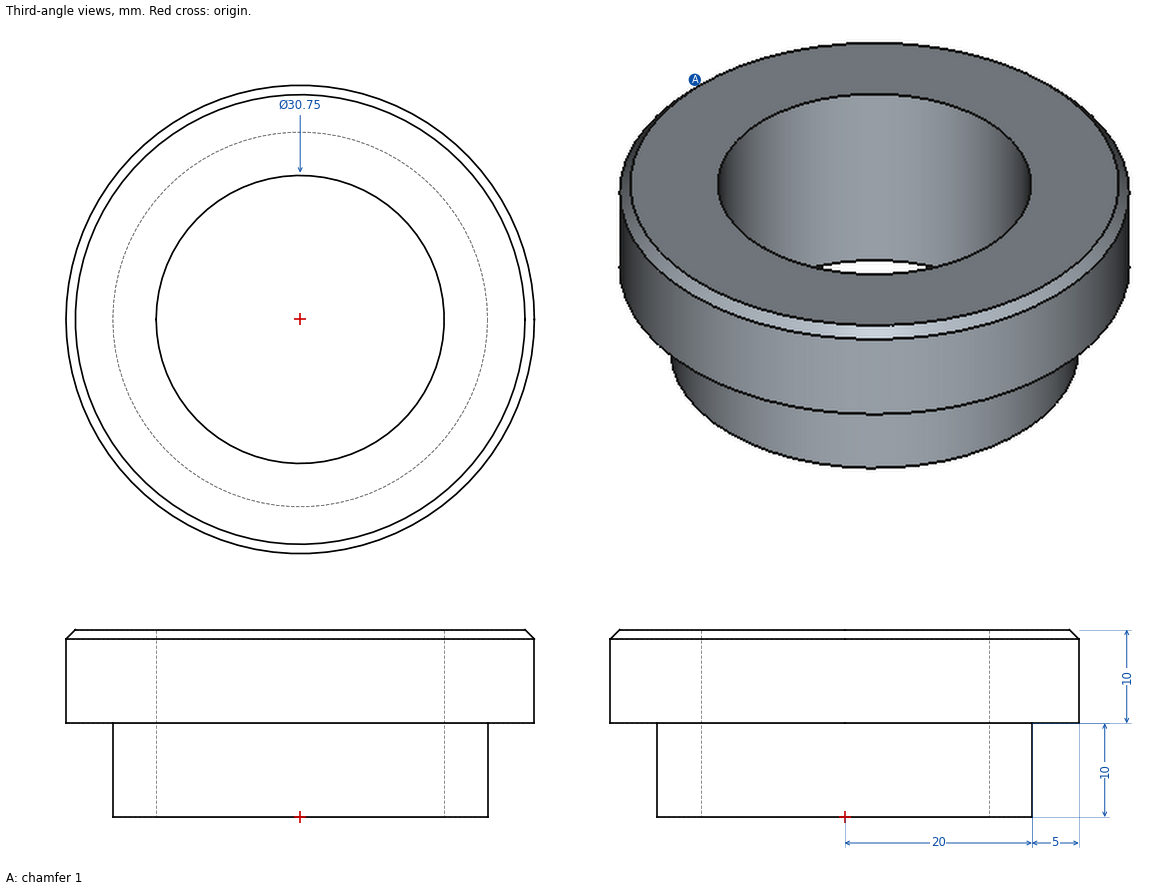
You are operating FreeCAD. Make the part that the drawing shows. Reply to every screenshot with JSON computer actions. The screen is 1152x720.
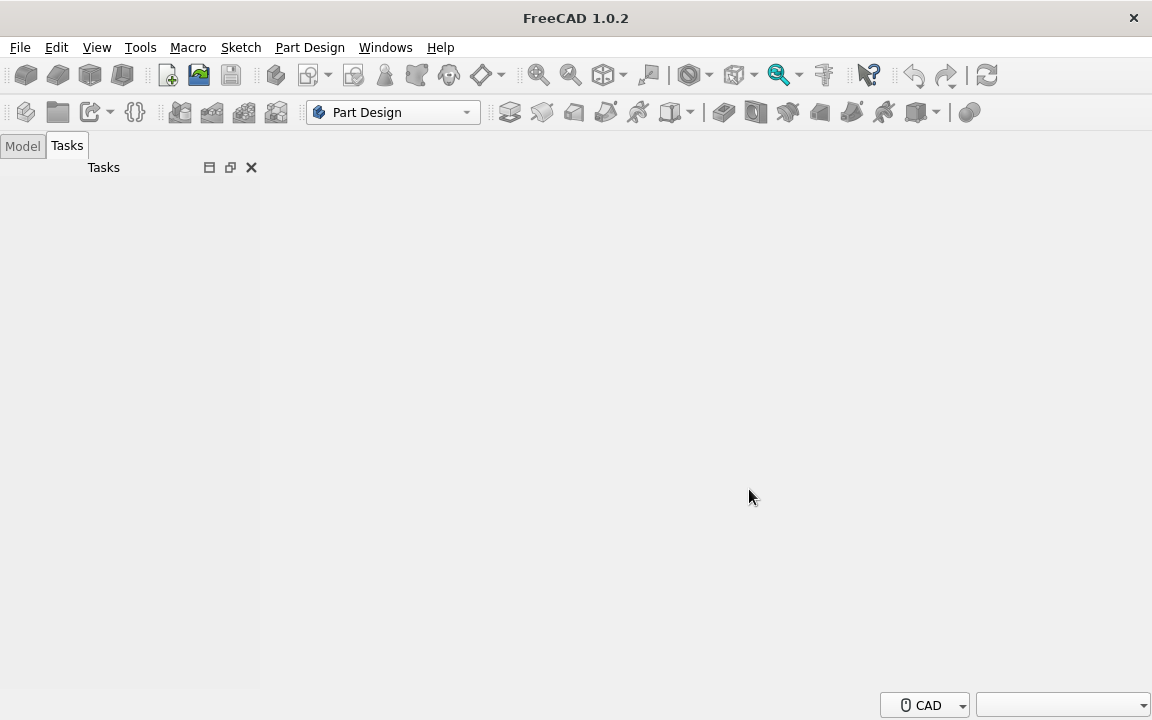
{"action": "key", "text": "ctrl+n"}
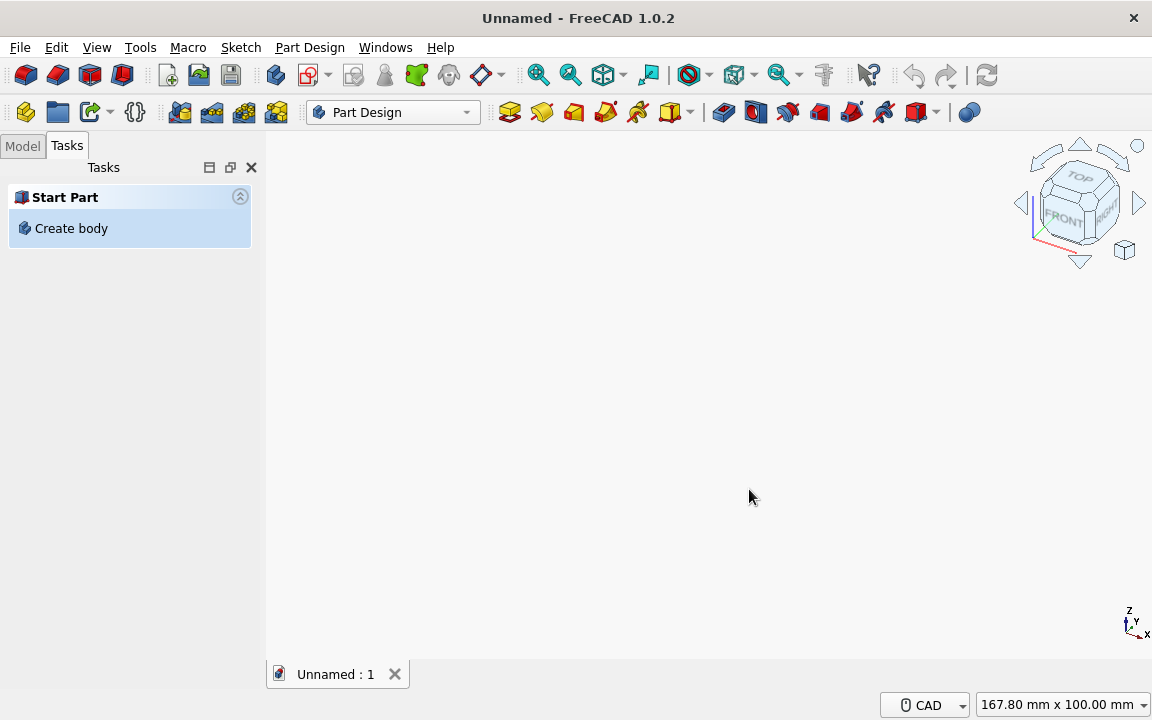
{"action": "left_click", "coordinate": [308, 76]}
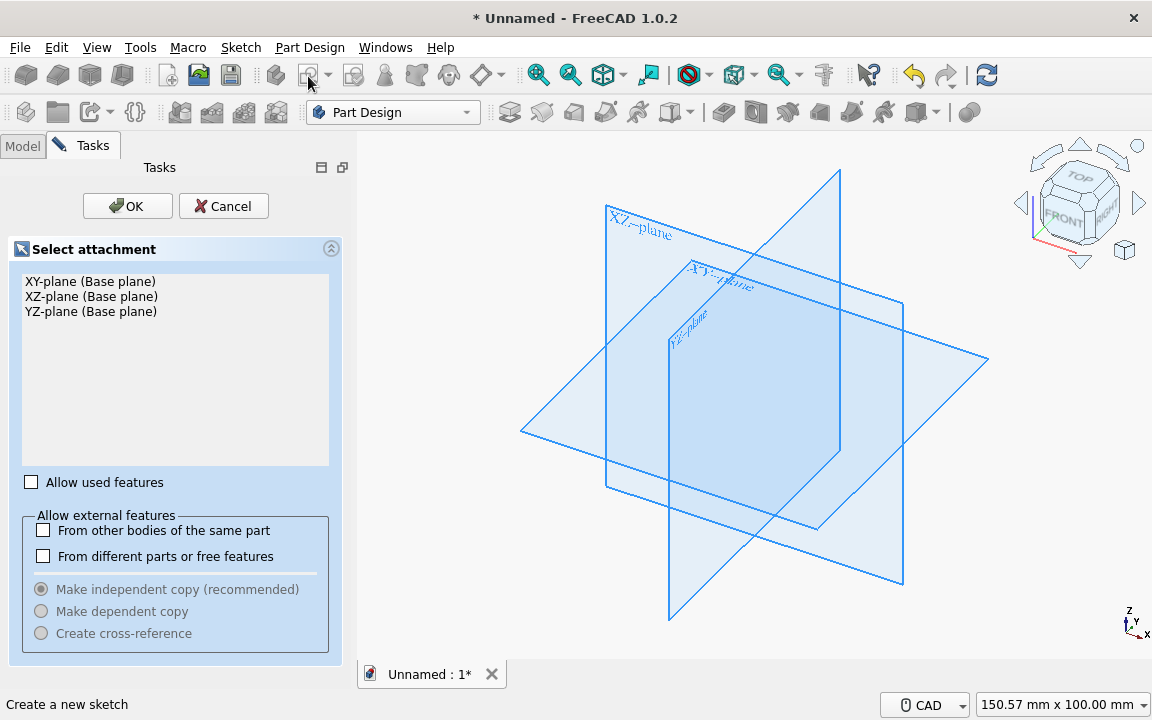
{"action": "left_click", "coordinate": [82, 312]}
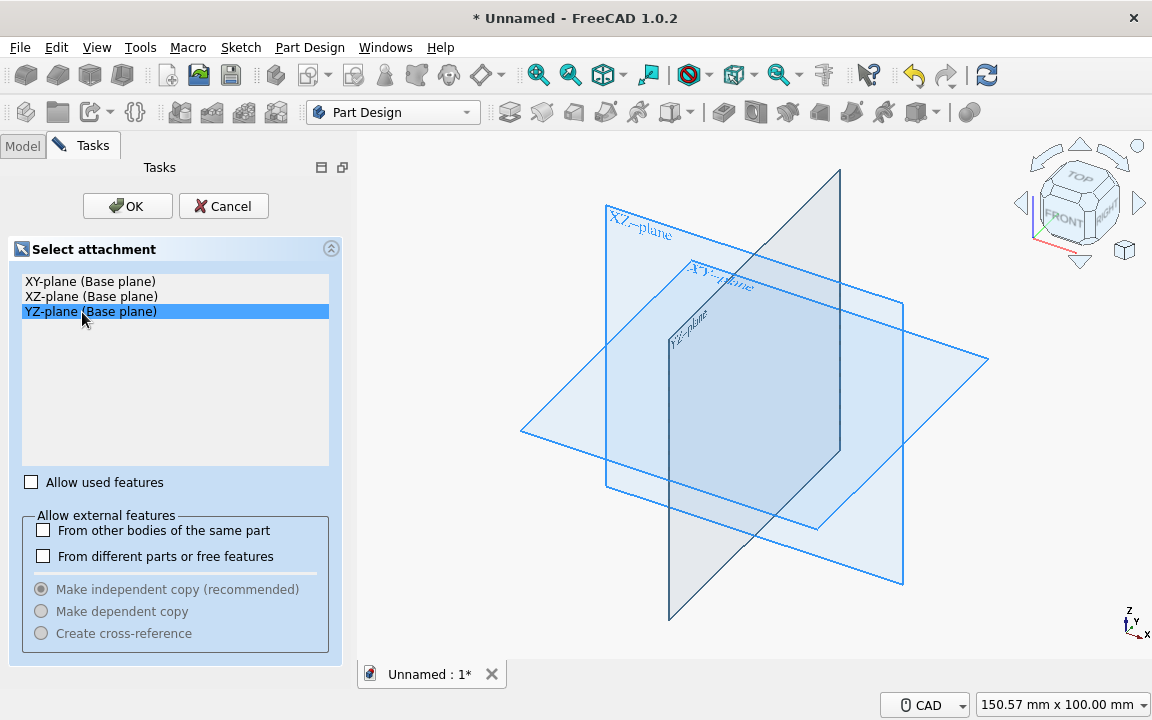
{"action": "left_click", "coordinate": [128, 206]}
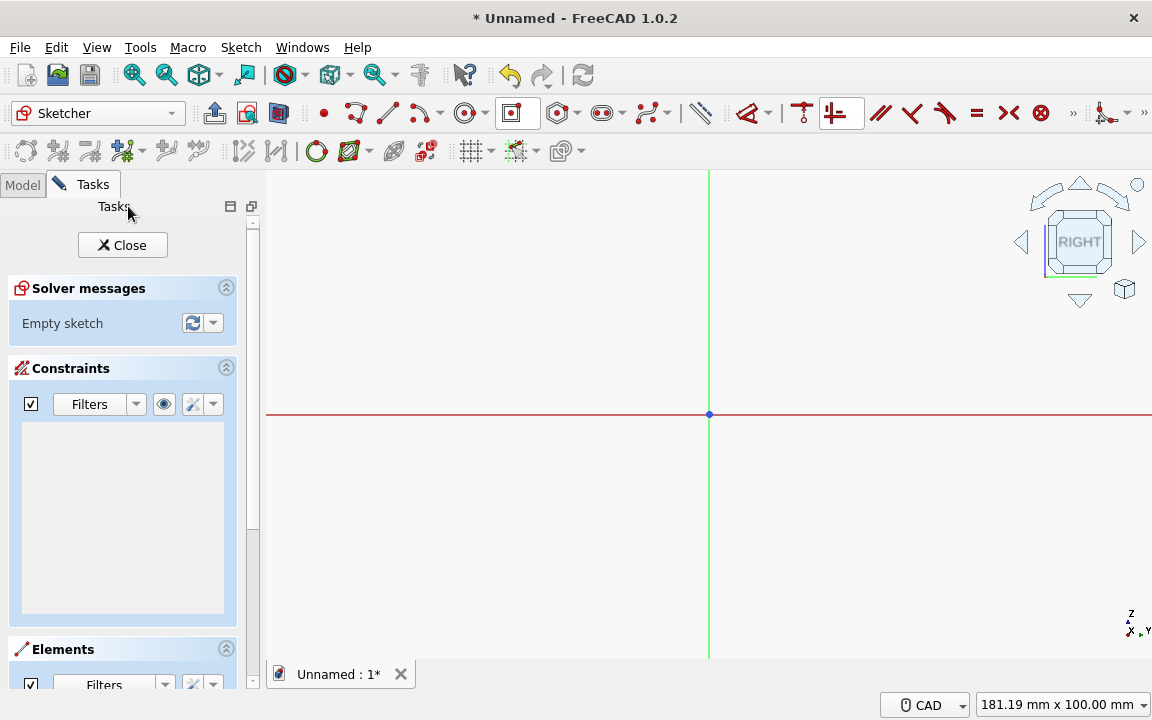
{"action": "scroll", "coordinate": [826, 345], "scroll_direction": "up", "scroll_amount": 6}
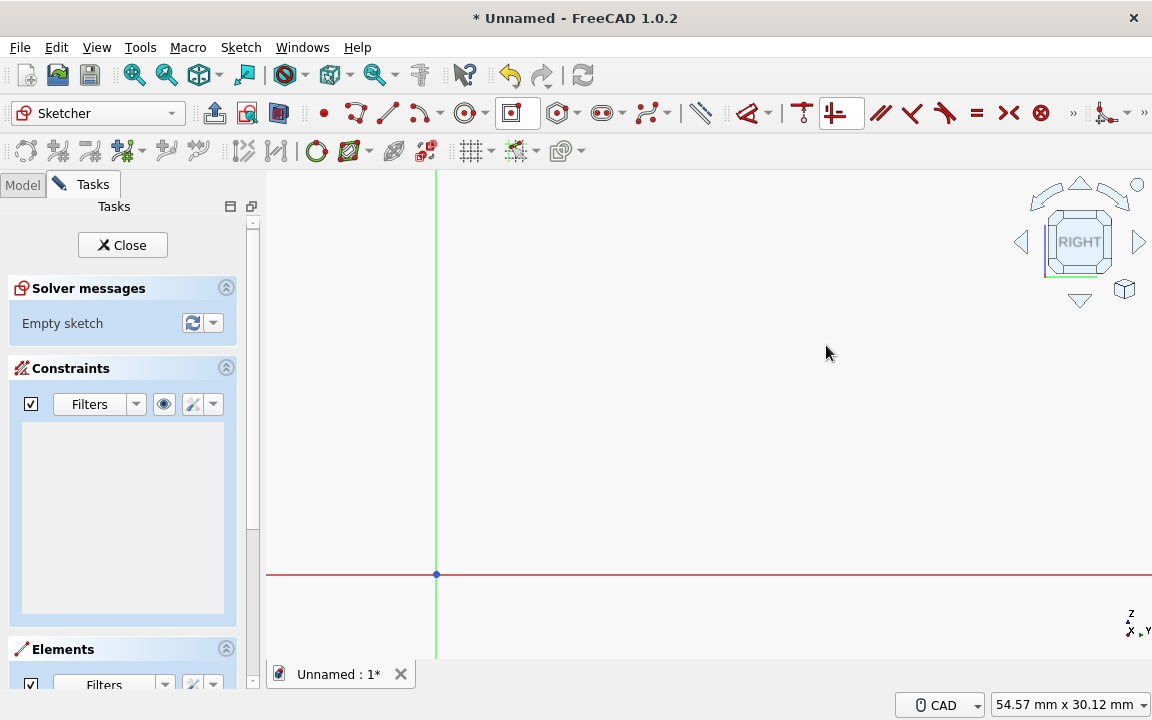
{"action": "left_click", "coordinate": [356, 114]}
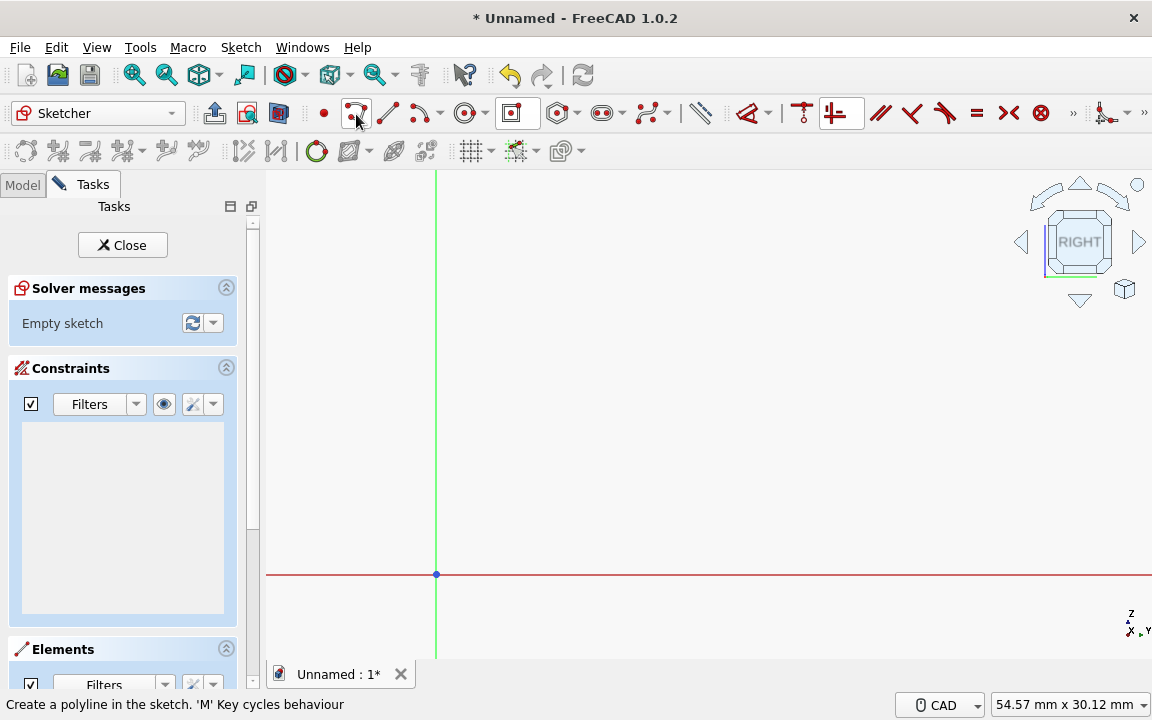
{"action": "left_click", "coordinate": [436, 575]}
{"action": "left_click", "coordinate": [761, 566]}
{"action": "left_click", "coordinate": [761, 413]}
{"action": "left_click", "coordinate": [842, 413]}
{"action": "left_click", "coordinate": [842, 250]}
{"action": "left_click", "coordinate": [445, 250]}
{"action": "left_click", "coordinate": [436, 575]}
{"action": "key", "text": "Escape"}
{"action": "key", "text": "Escape"}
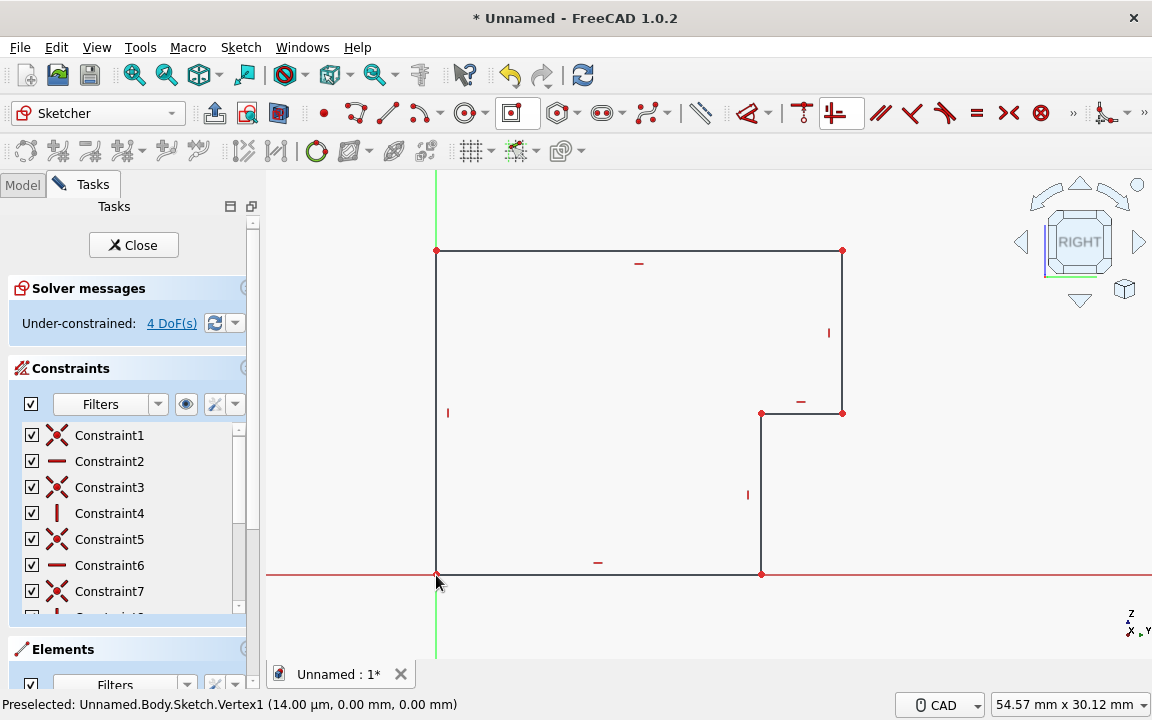
{"action": "left_click", "coordinate": [785, 414]}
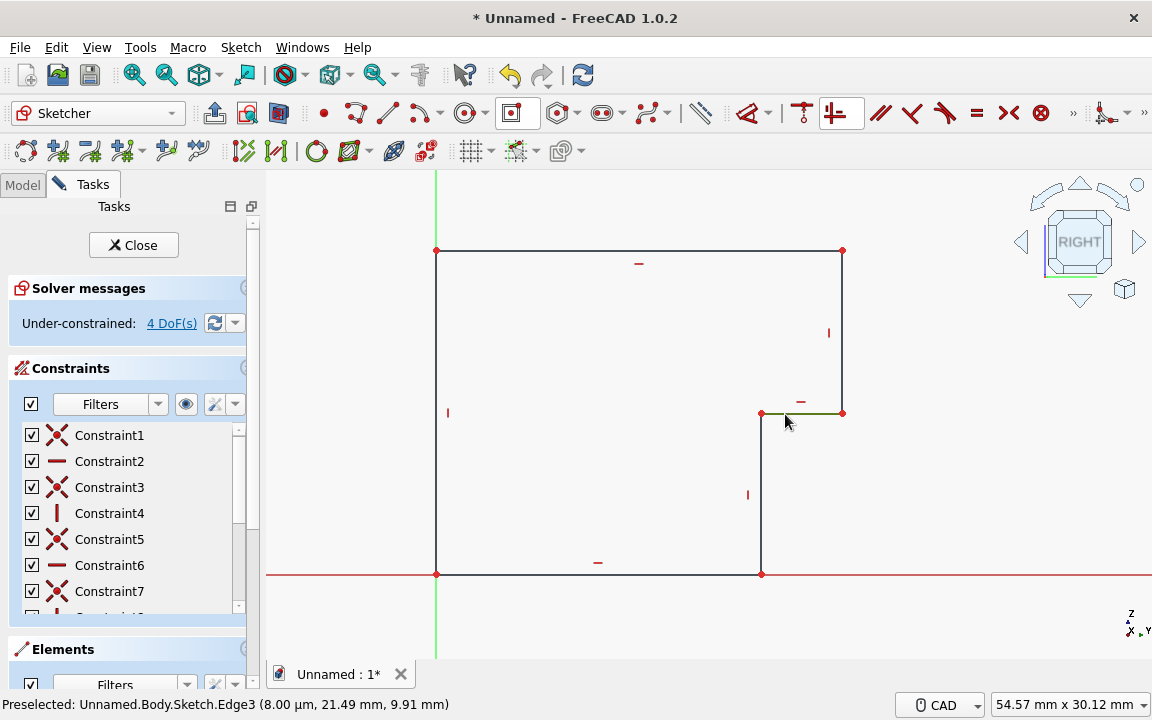
{"action": "key", "text": "l"}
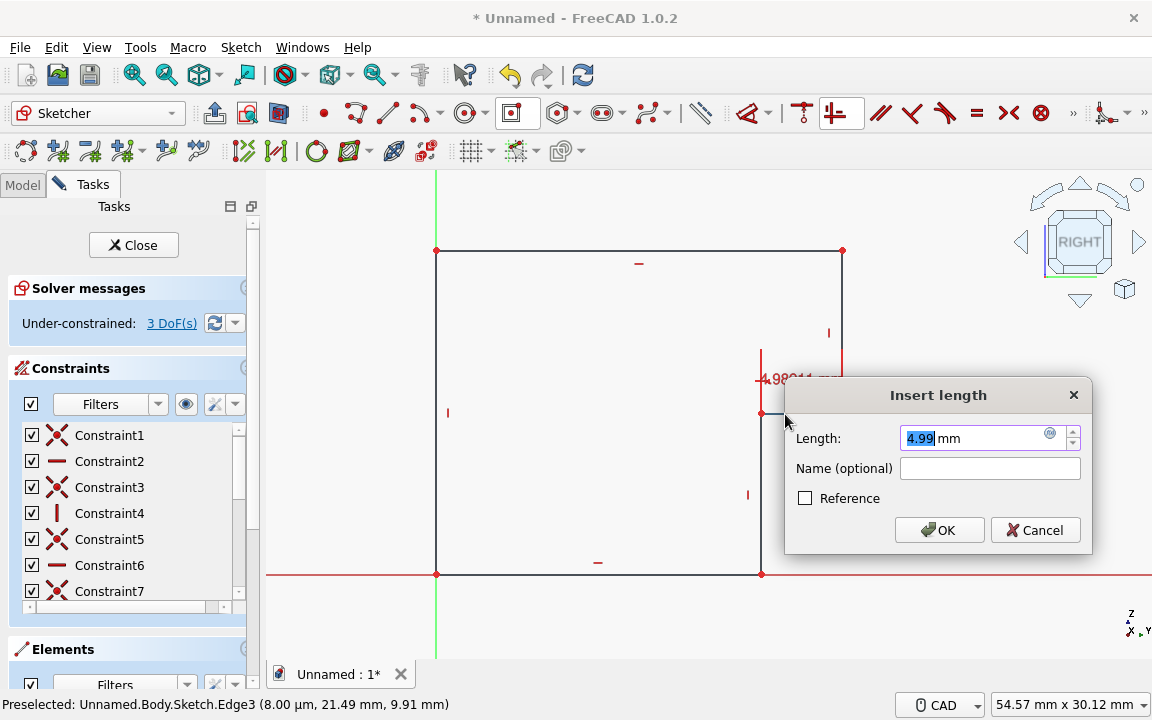
{"action": "type", "text": "5"}
{"action": "key", "text": "Return"}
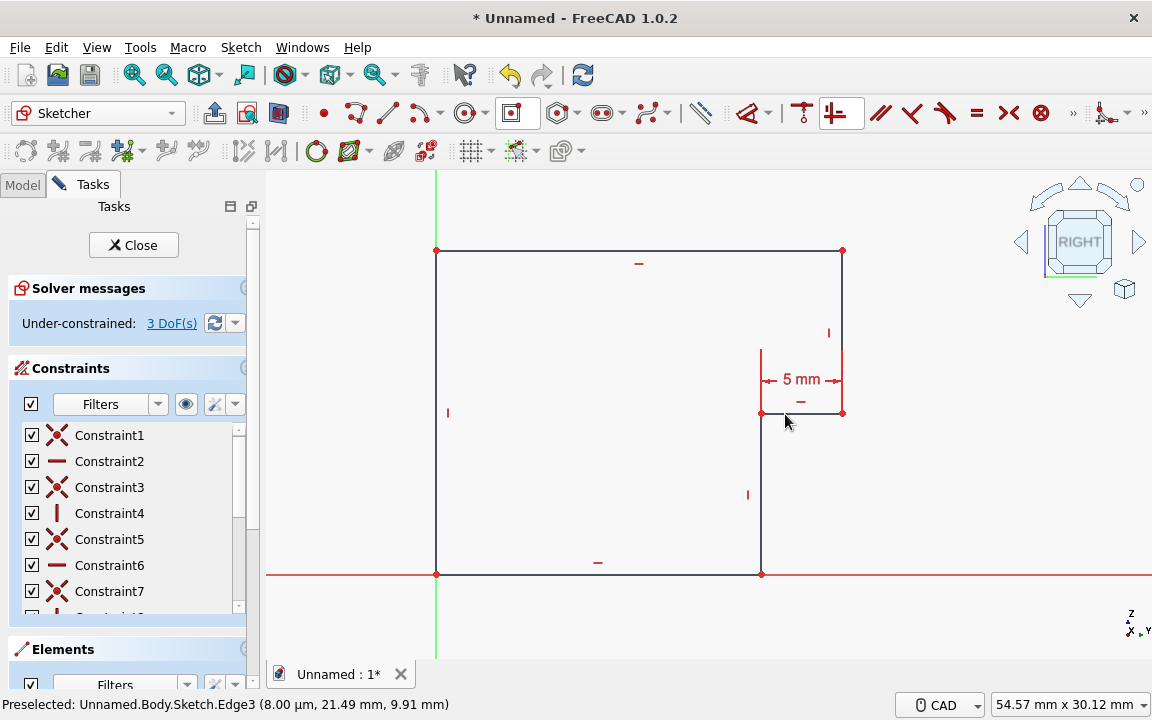
{"action": "left_click", "coordinate": [534, 575]}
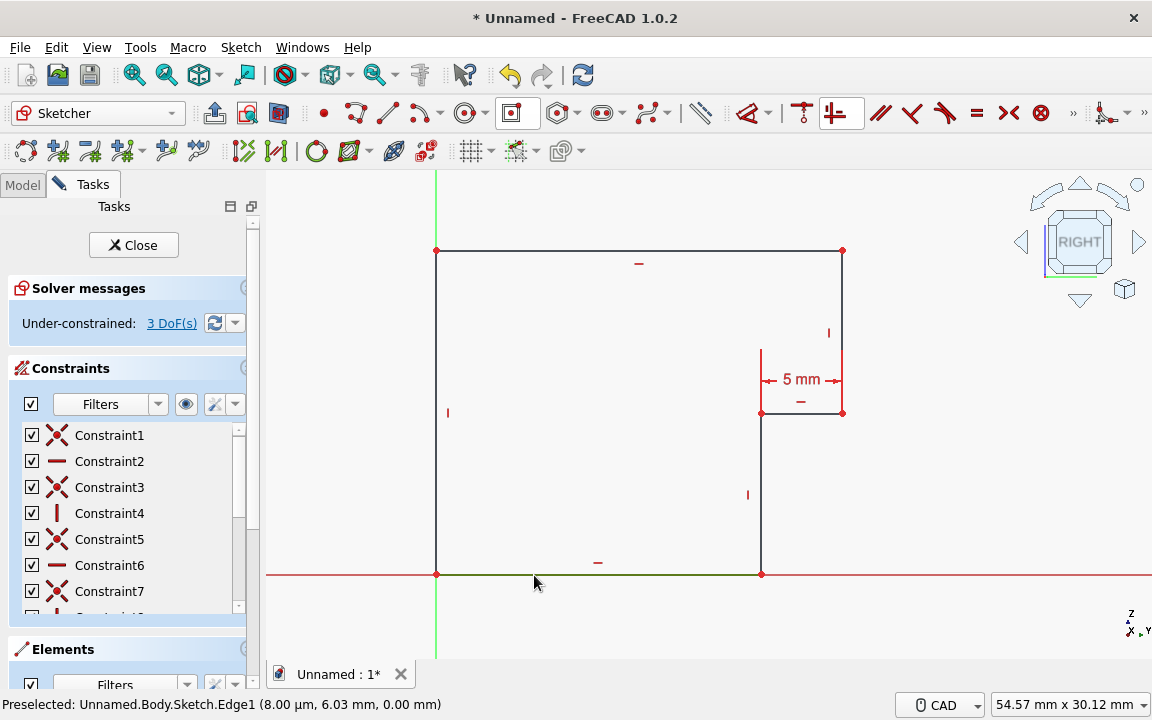
{"action": "key", "text": "l"}